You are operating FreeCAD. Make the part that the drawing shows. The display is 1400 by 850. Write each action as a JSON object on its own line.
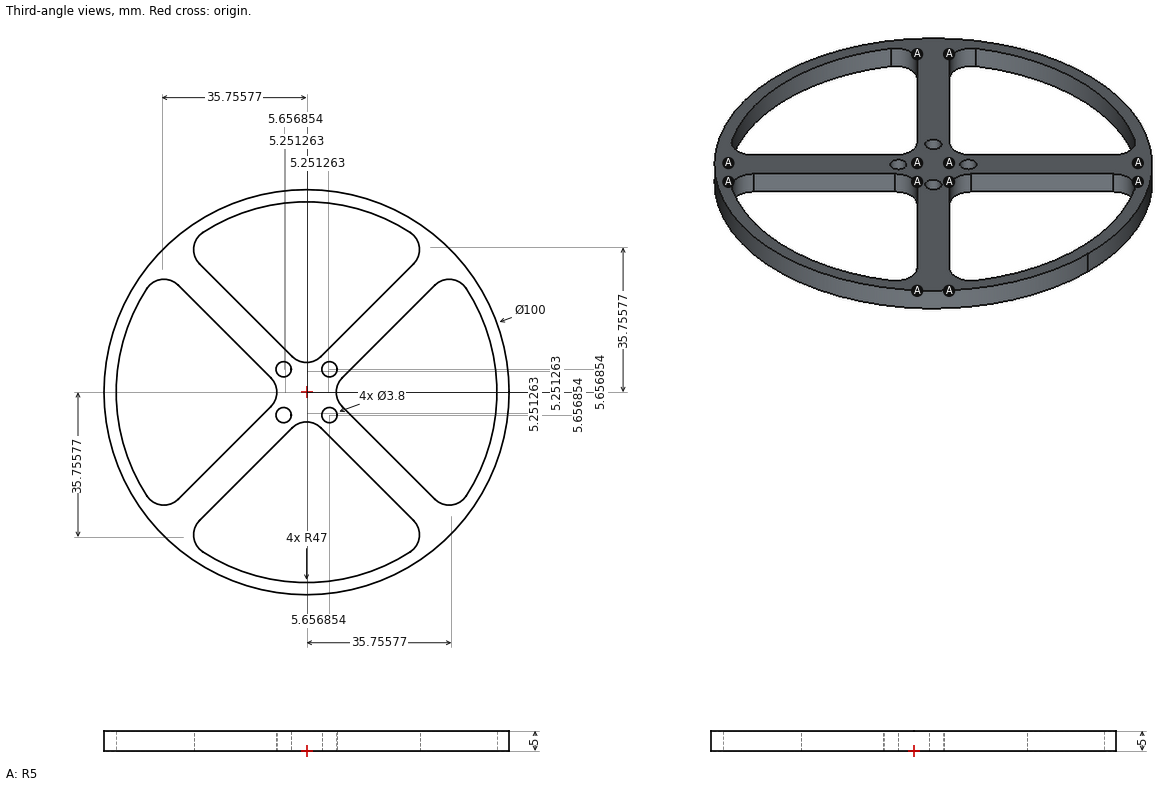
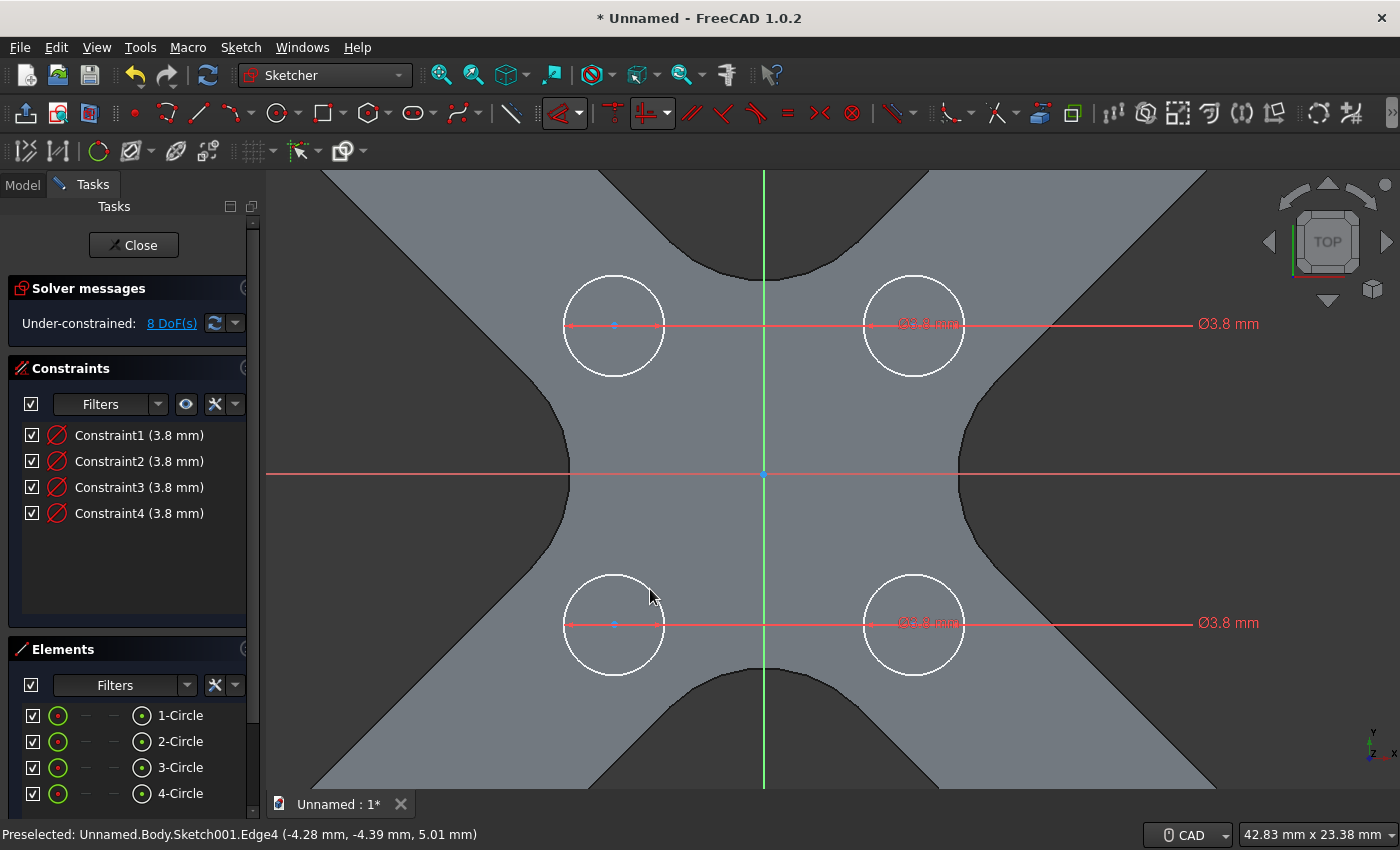
{"action": "left_click", "coordinate": [914, 625]}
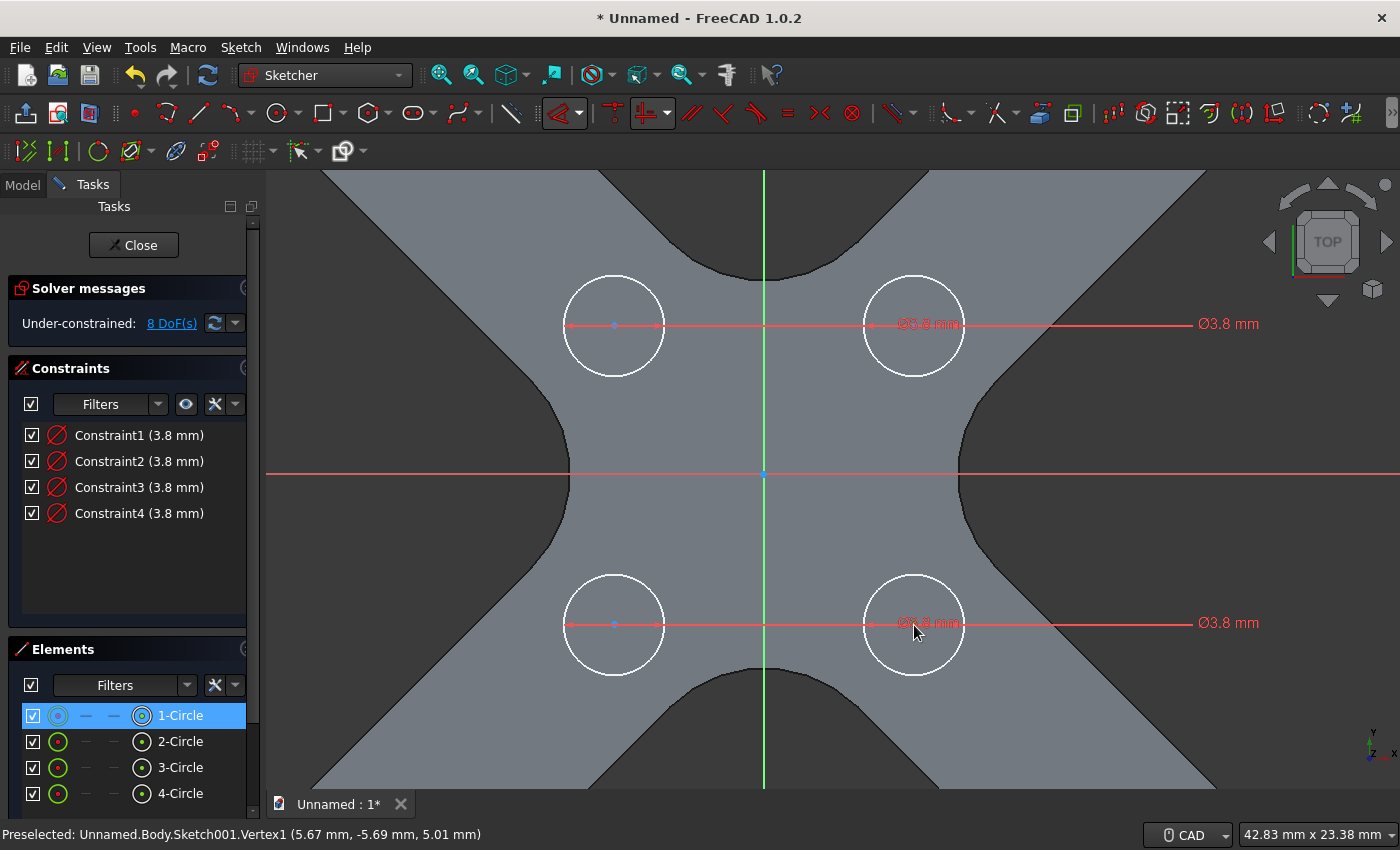
{"action": "left_click", "coordinate": [914, 326]}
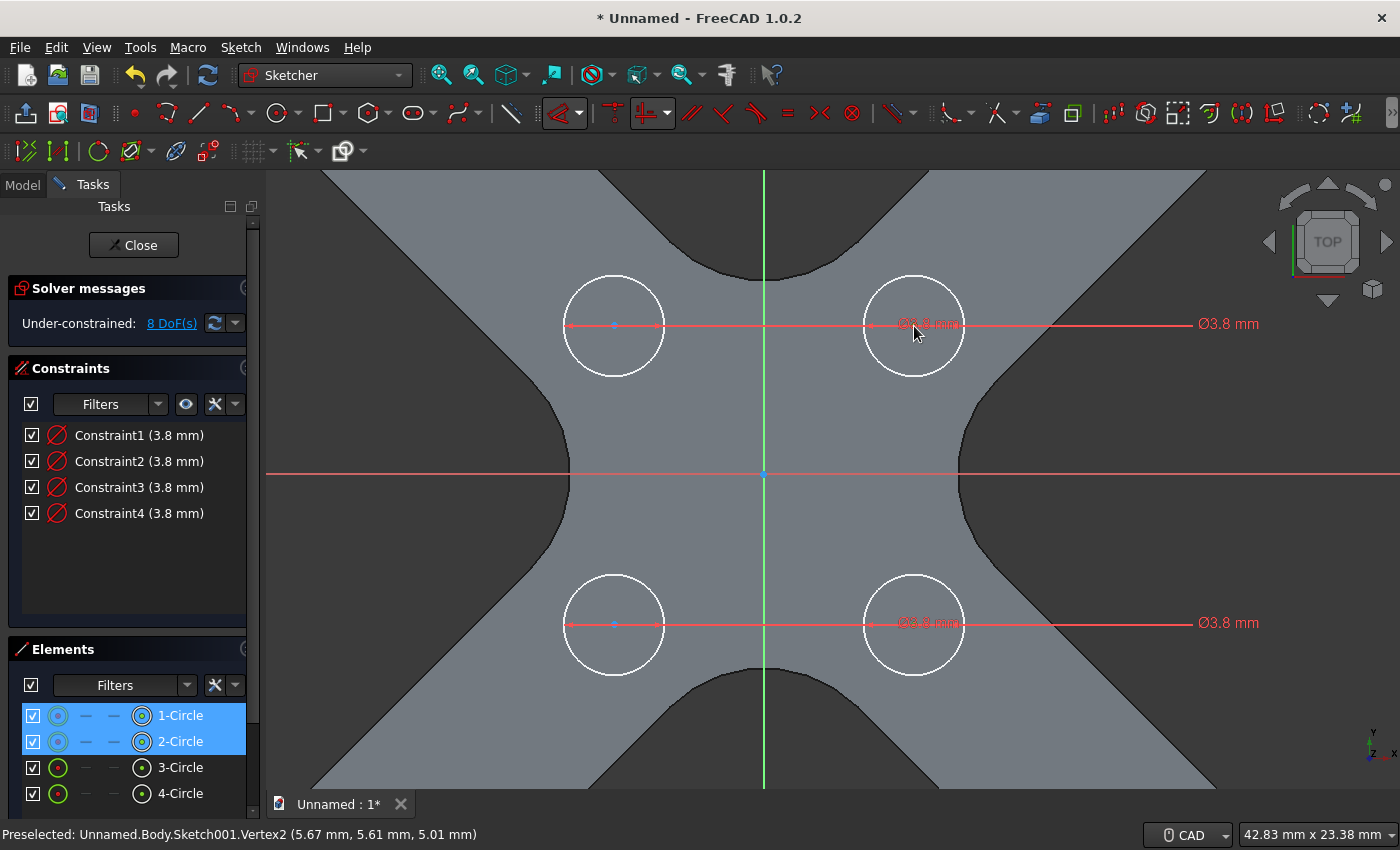
{"action": "left_click", "coordinate": [670, 114]}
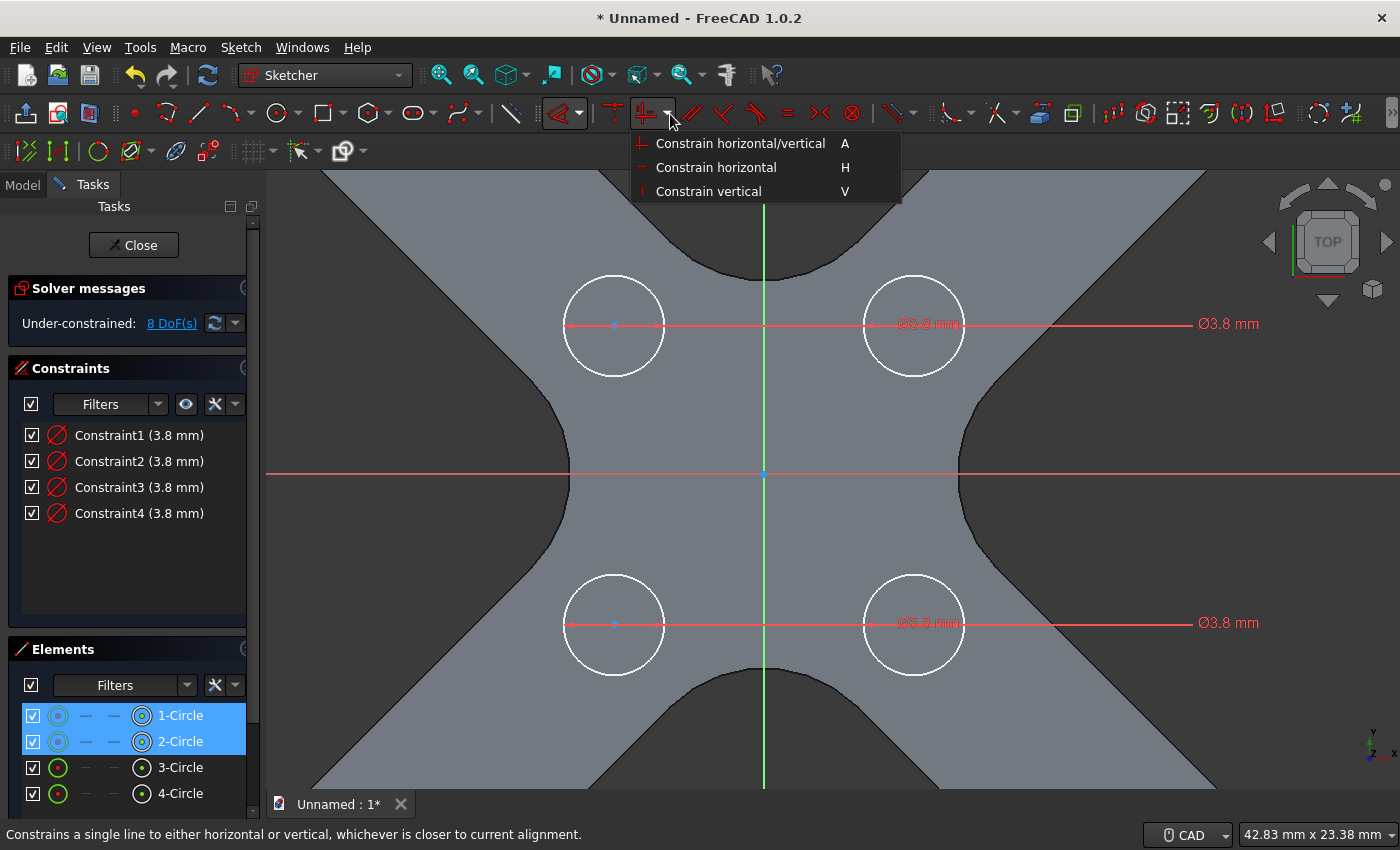
{"action": "left_click", "coordinate": [766, 191]}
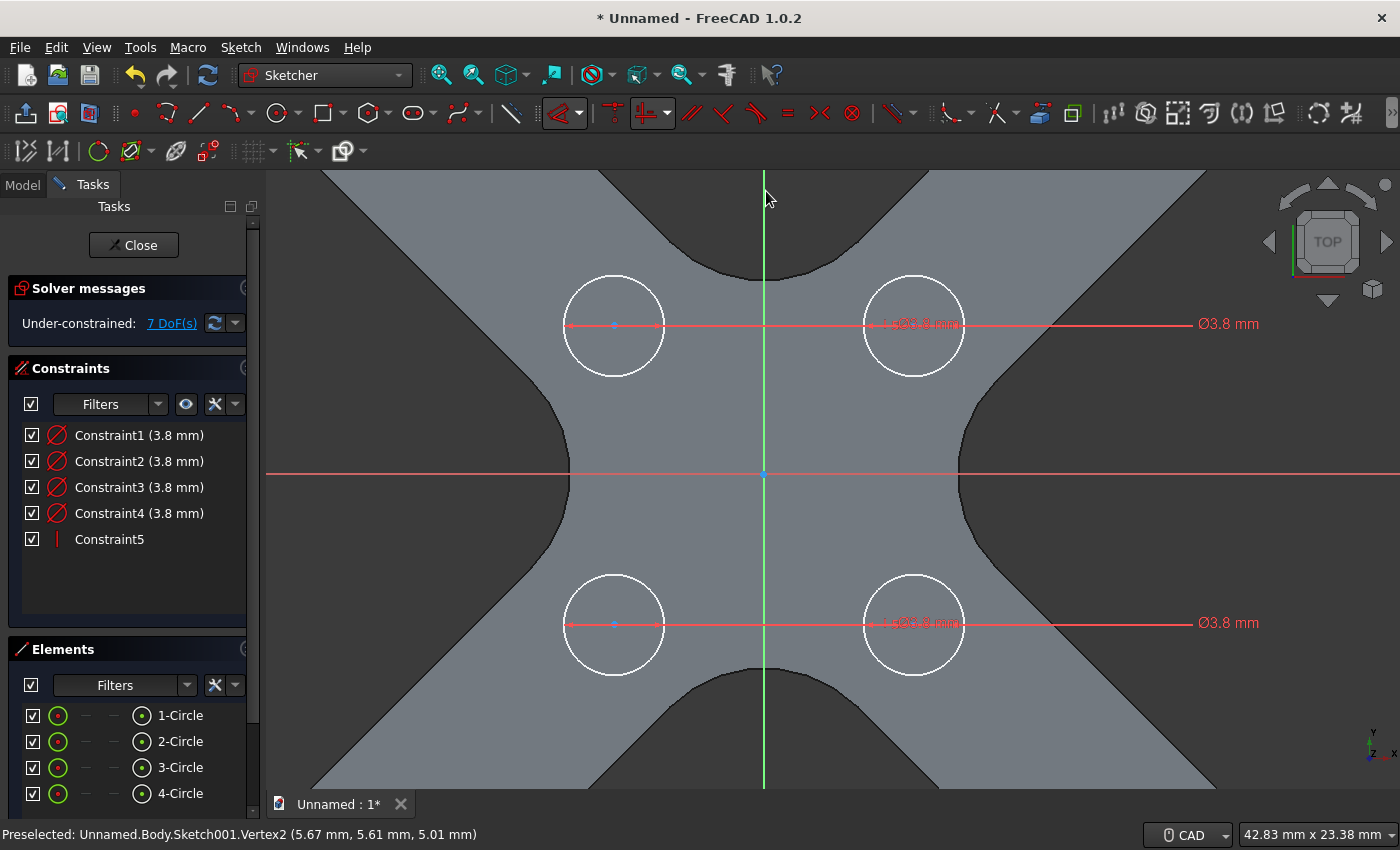
{"action": "left_click", "coordinate": [914, 326]}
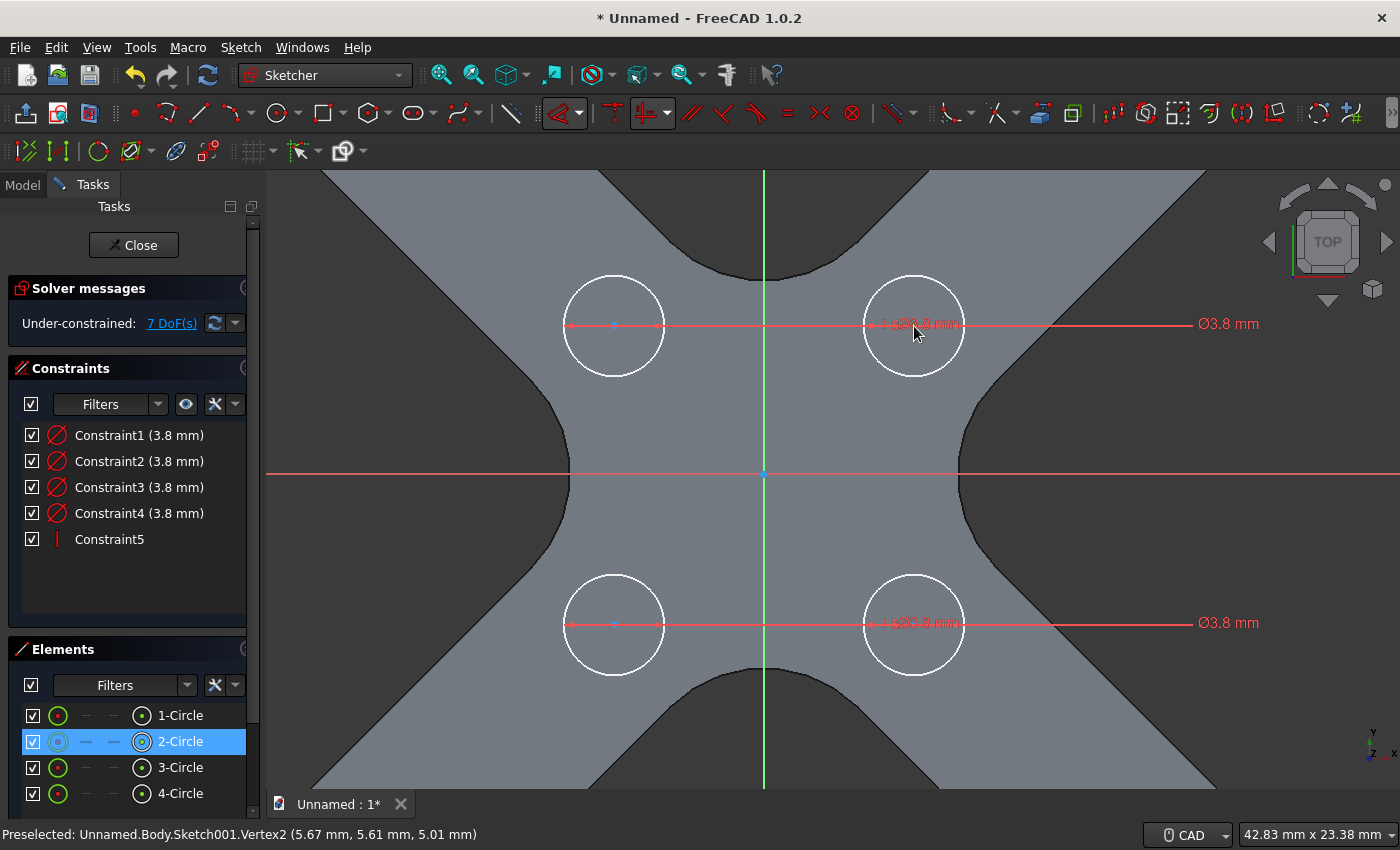
{"action": "left_click", "coordinate": [614, 326]}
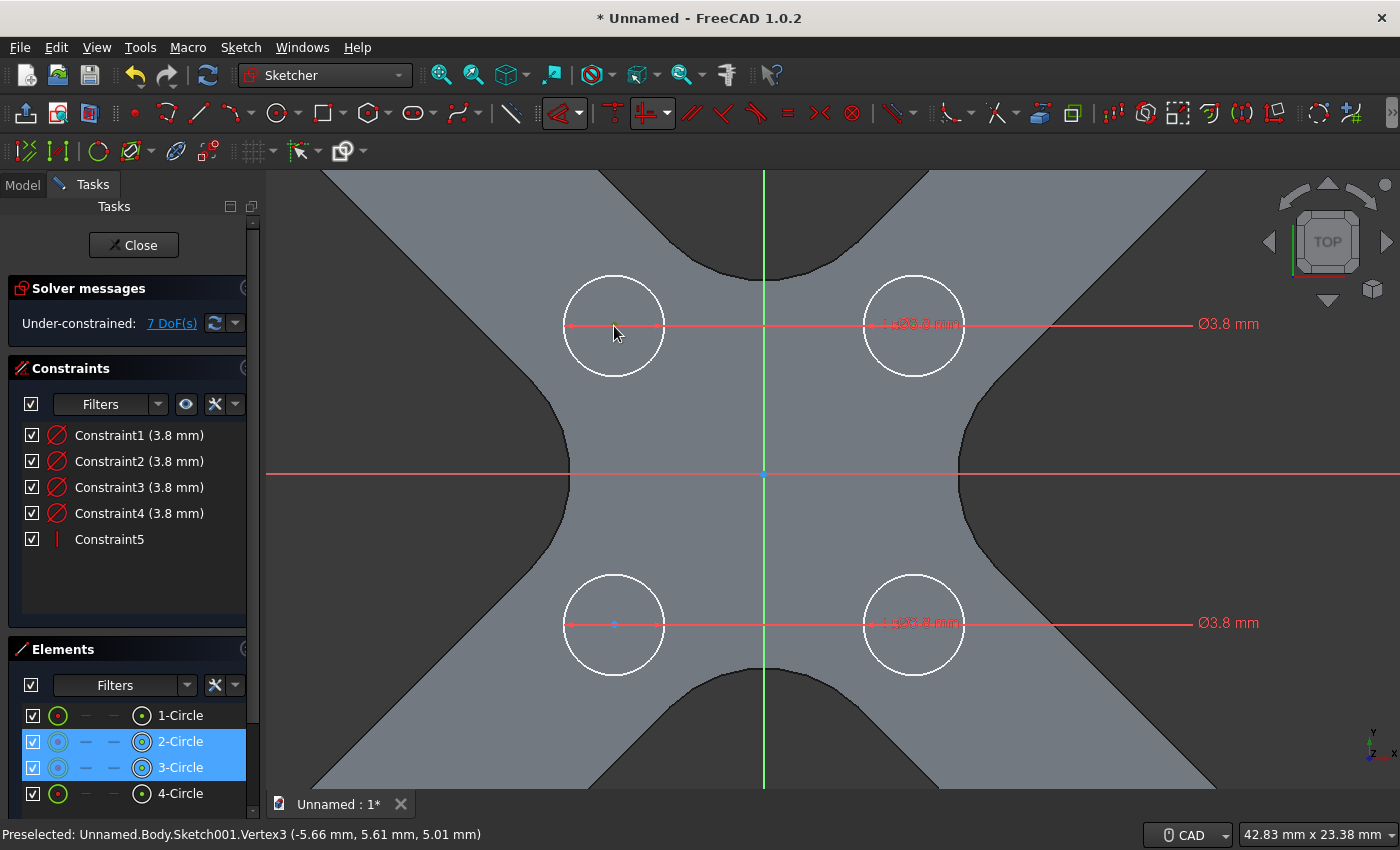
{"action": "key", "text": "h"}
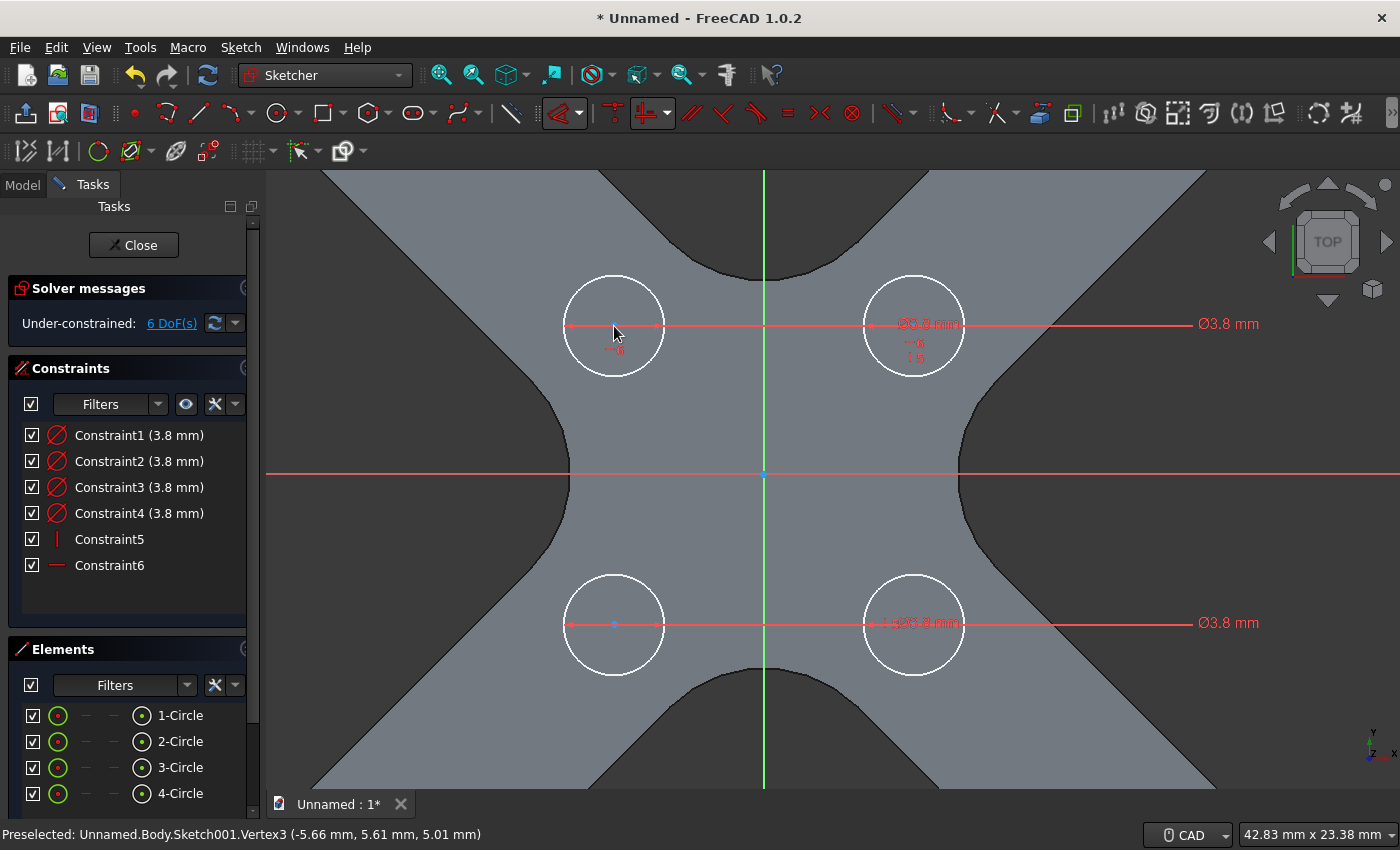
{"action": "left_click", "coordinate": [614, 326]}